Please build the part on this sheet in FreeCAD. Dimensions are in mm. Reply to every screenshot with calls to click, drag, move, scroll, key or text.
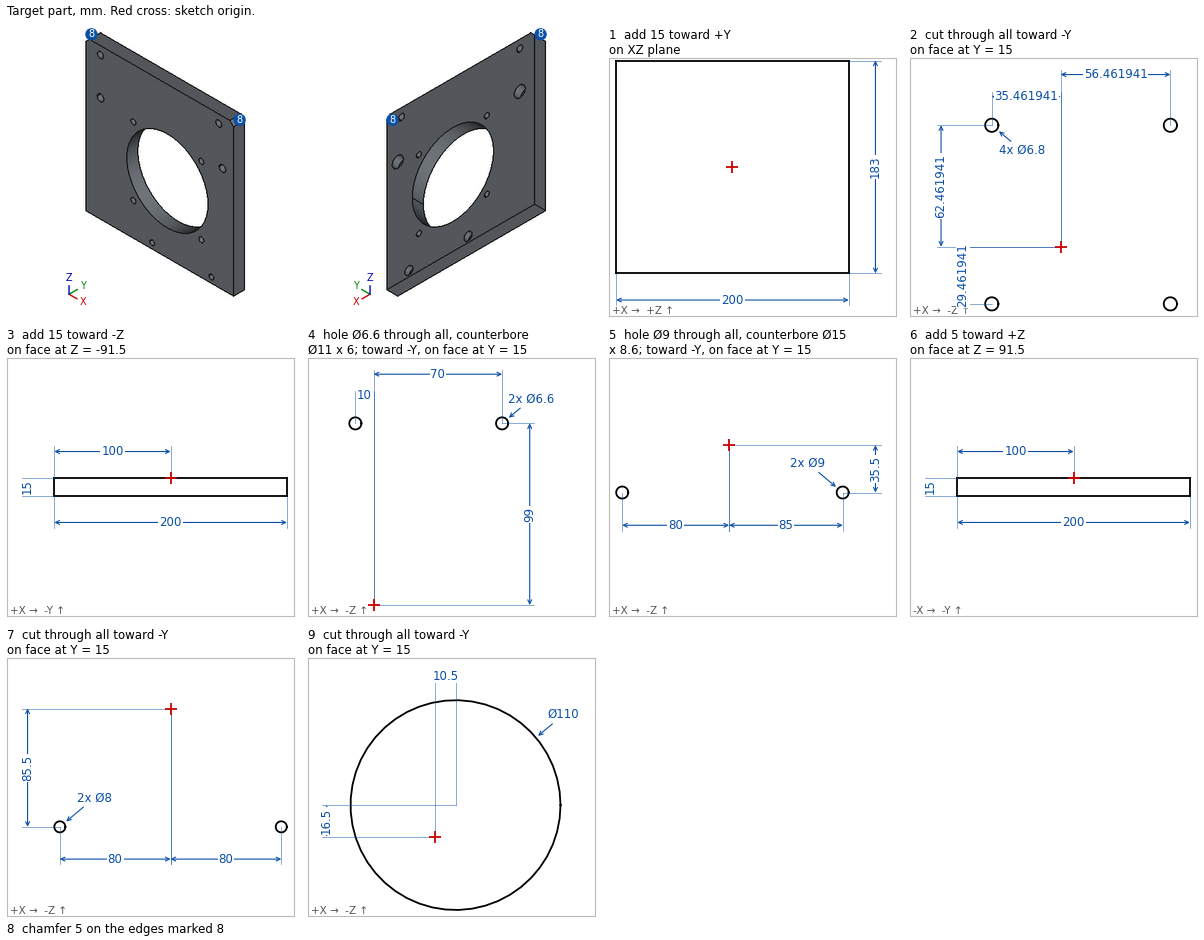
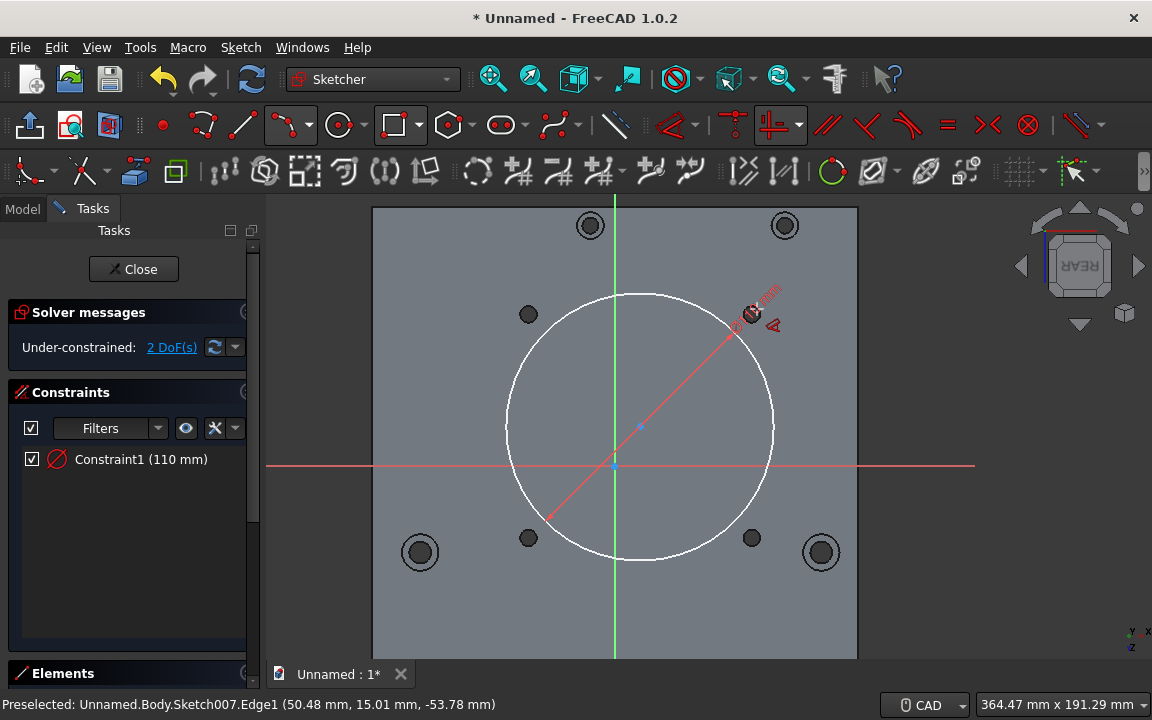
scroll(640, 427, up, 3)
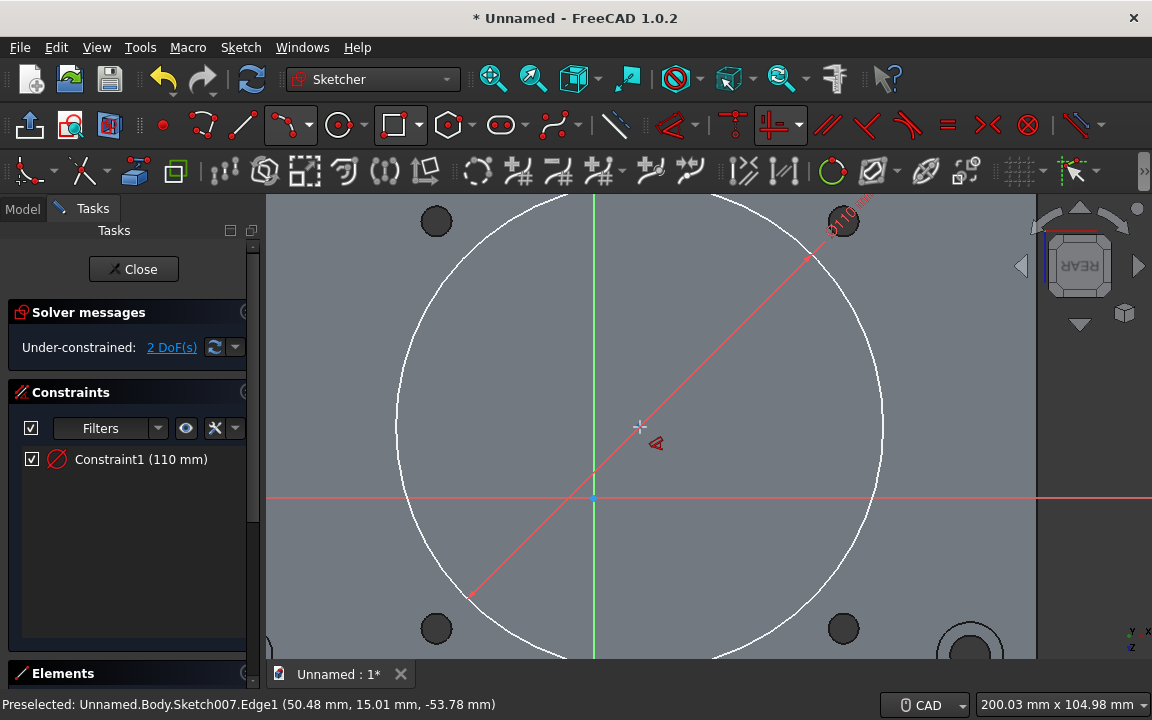
click(640, 427)
click(617, 532)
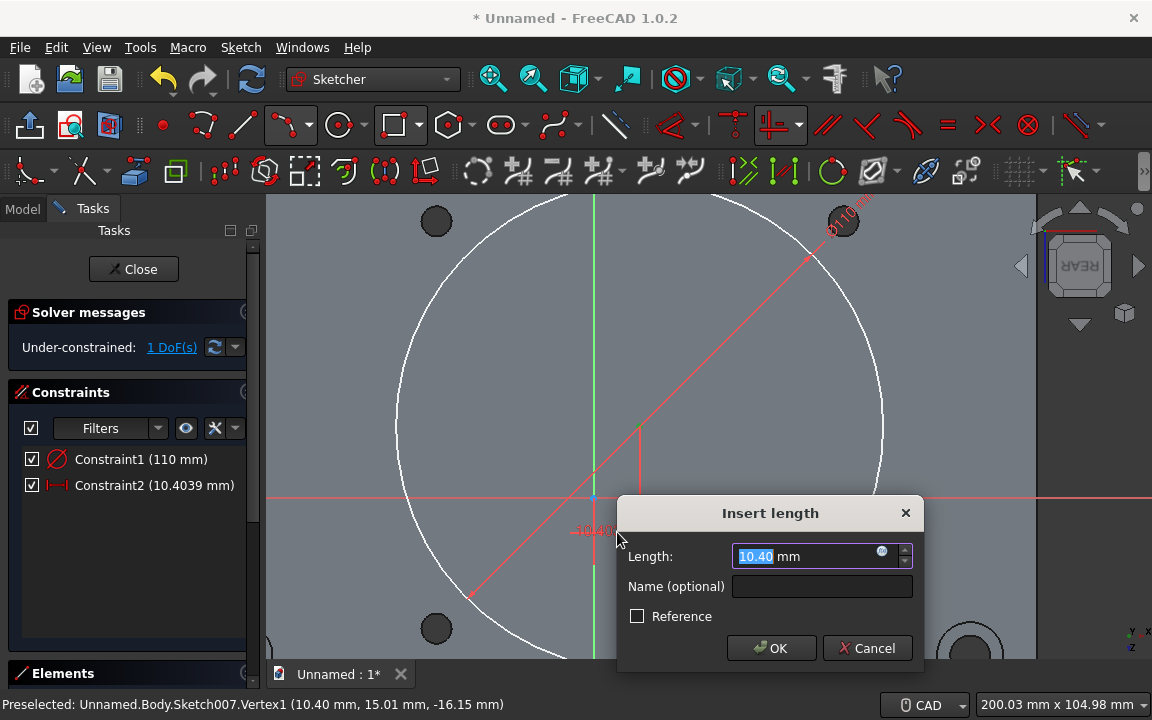
text(10.5)
key(Return)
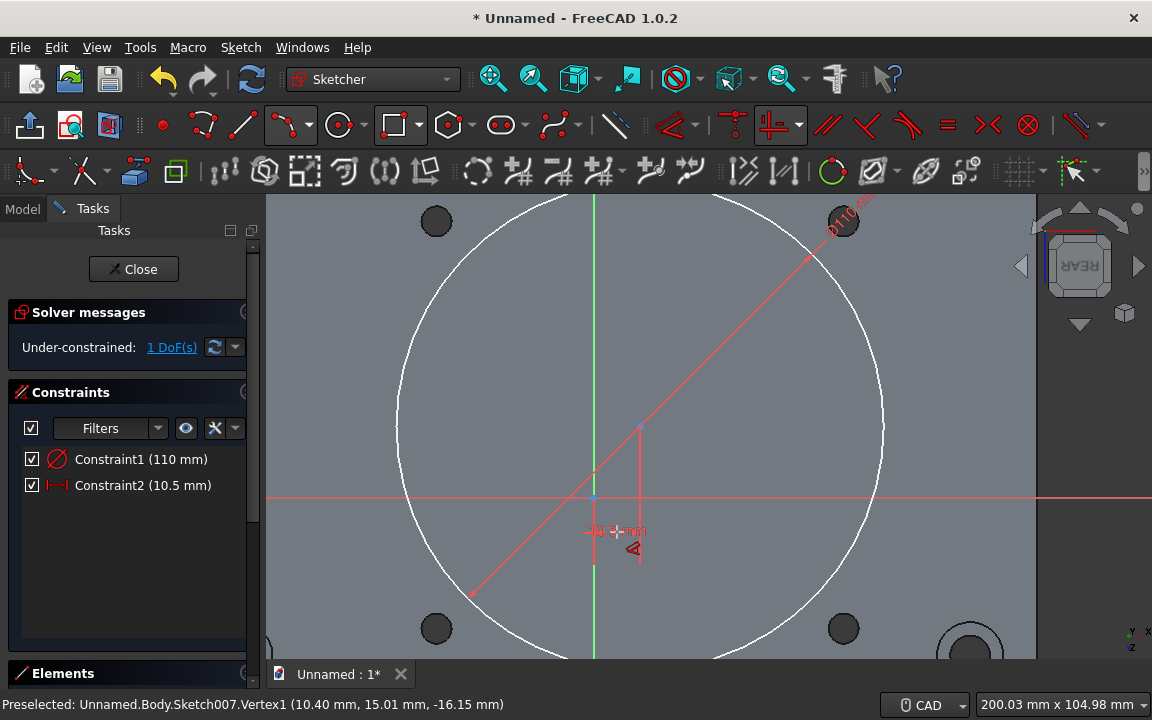
click(640, 427)
click(560, 462)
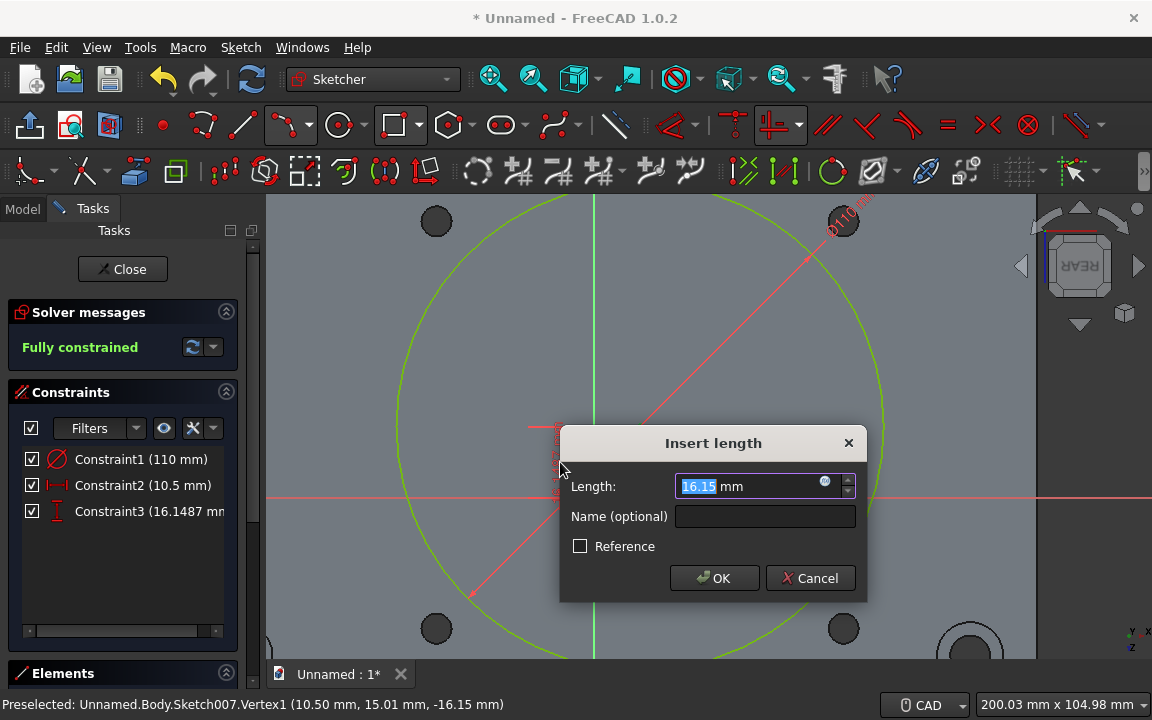
text(16.5)
key(Return)
key(Escape)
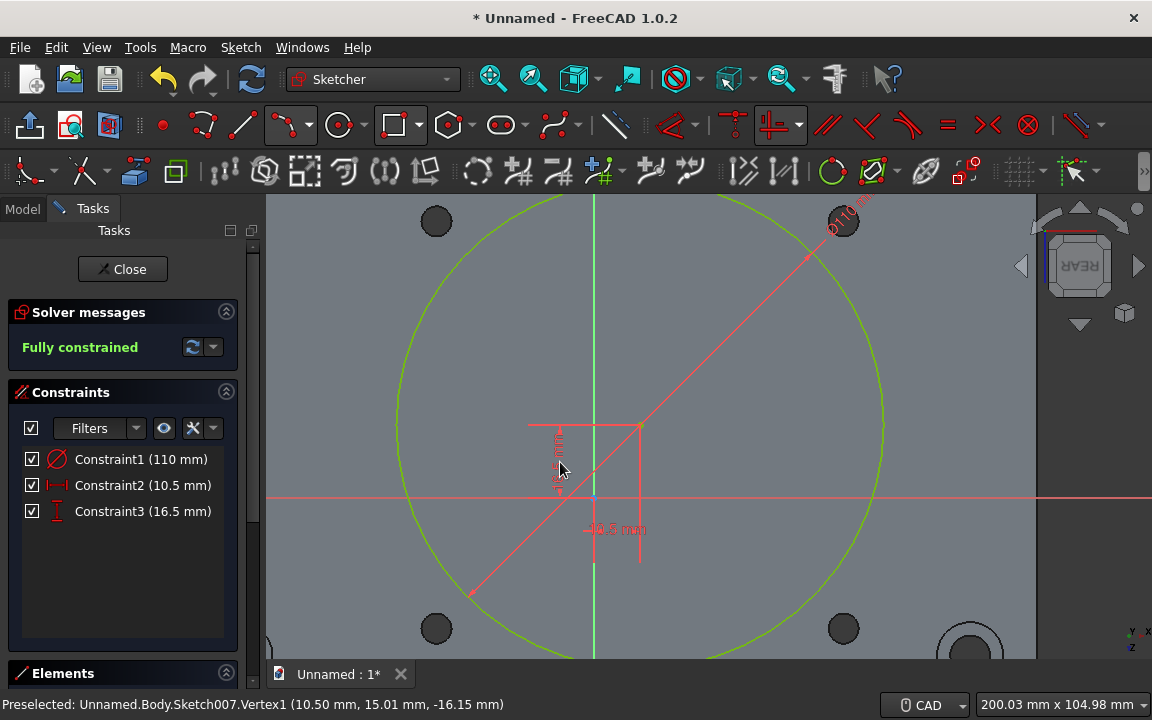
click(123, 269)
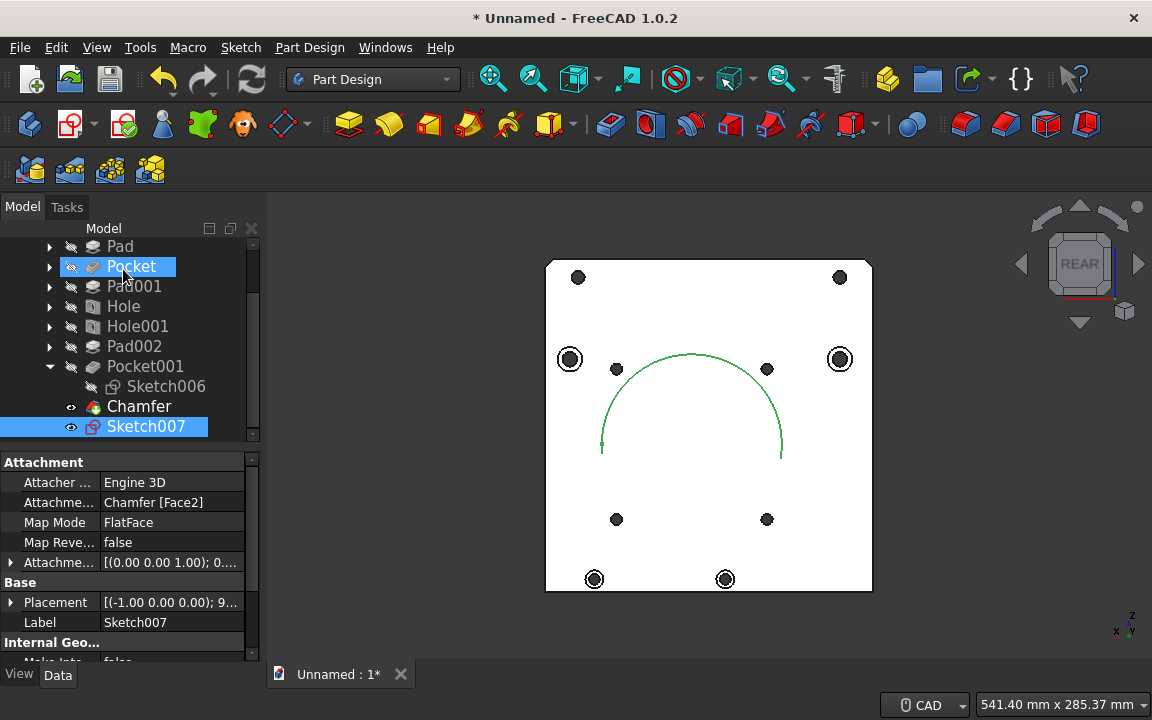
click(612, 124)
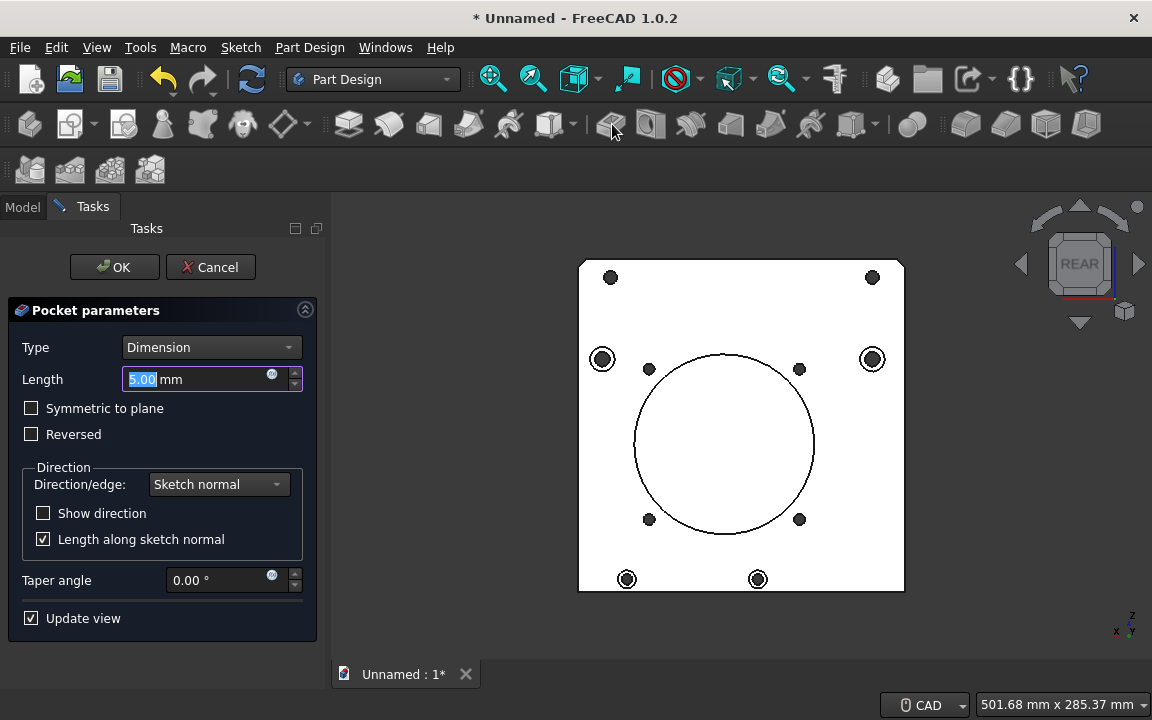
click(212, 348)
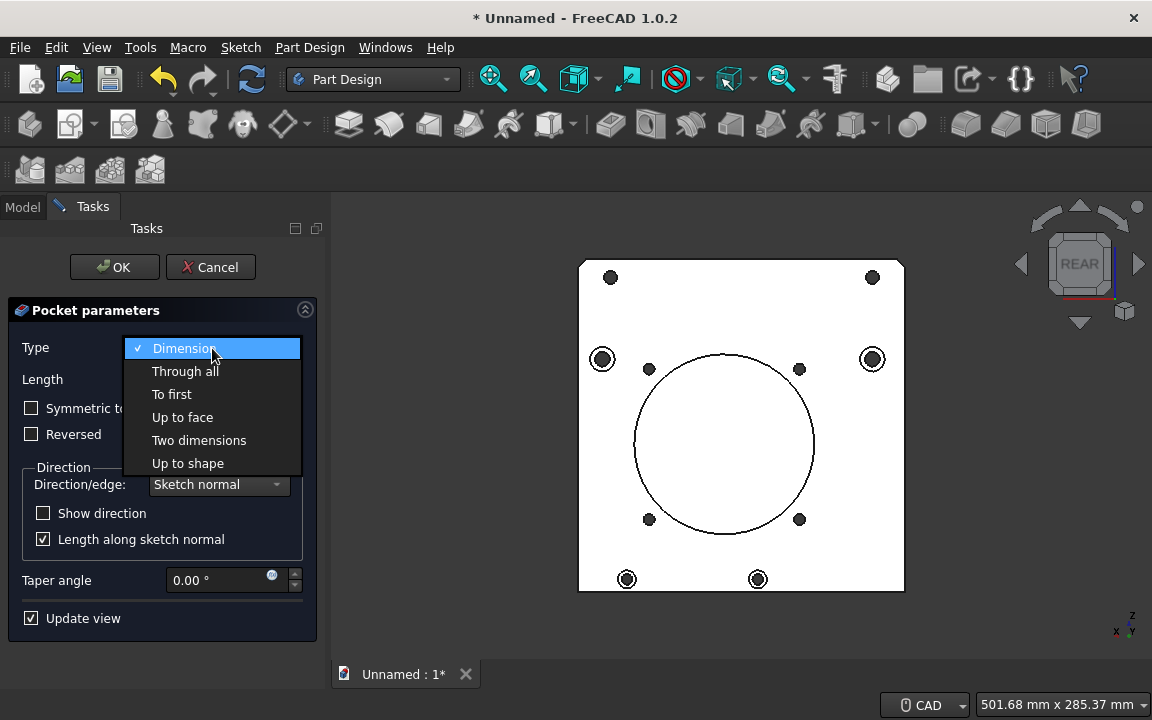
click(212, 372)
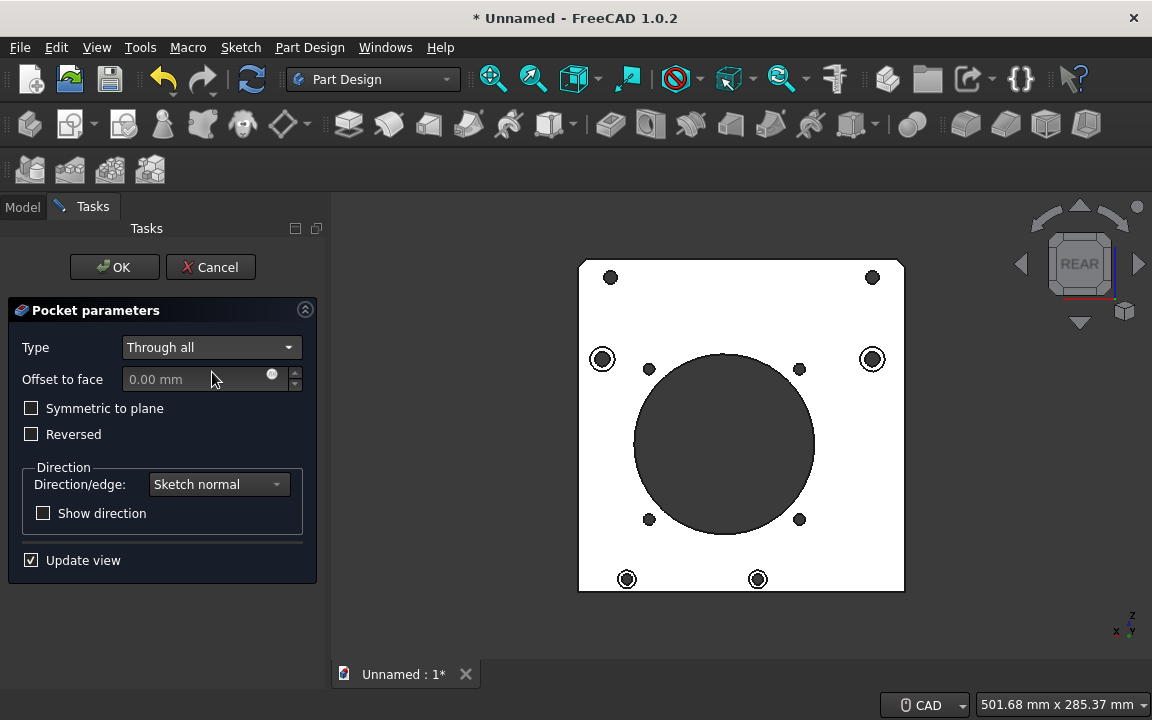
click(115, 267)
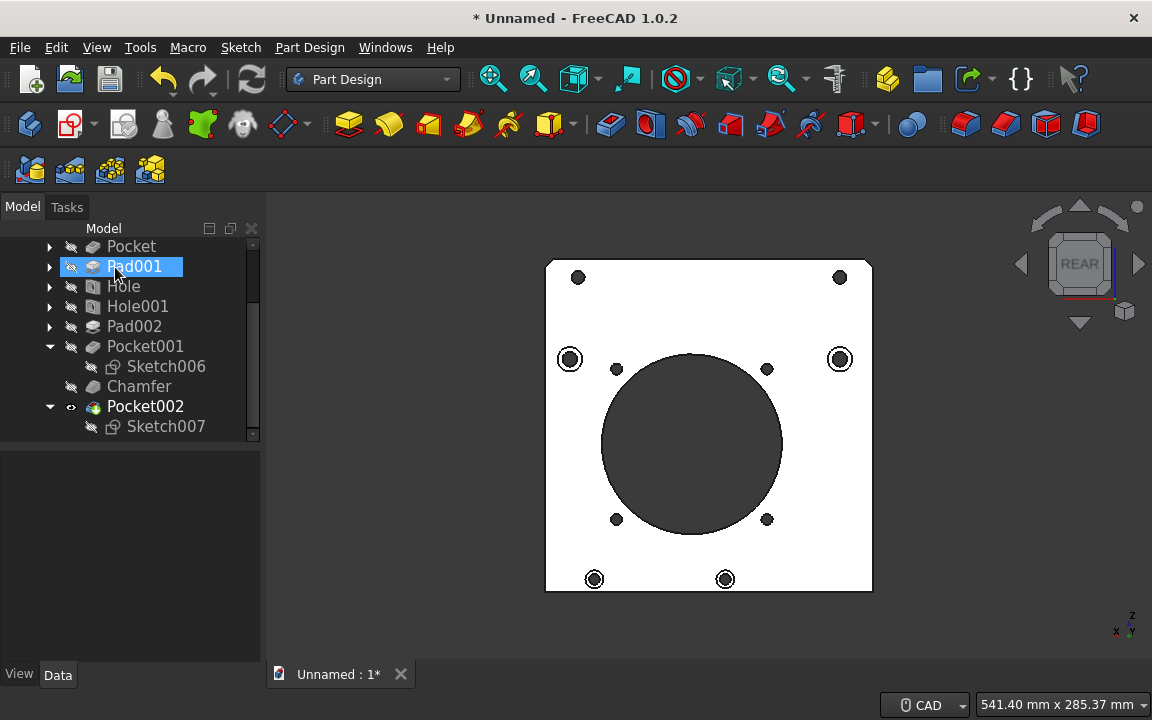
key(0)